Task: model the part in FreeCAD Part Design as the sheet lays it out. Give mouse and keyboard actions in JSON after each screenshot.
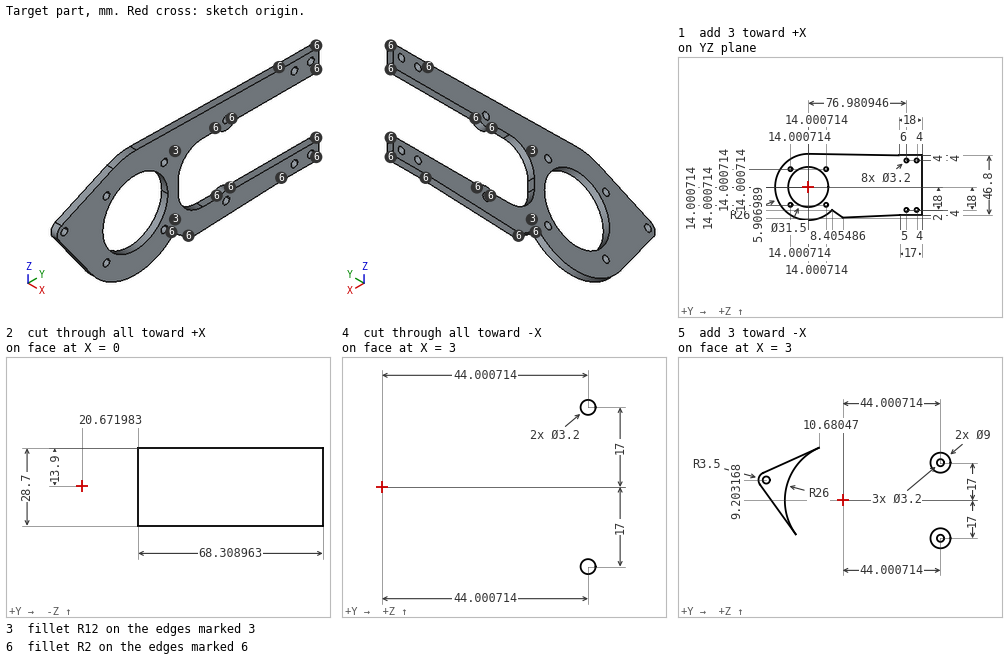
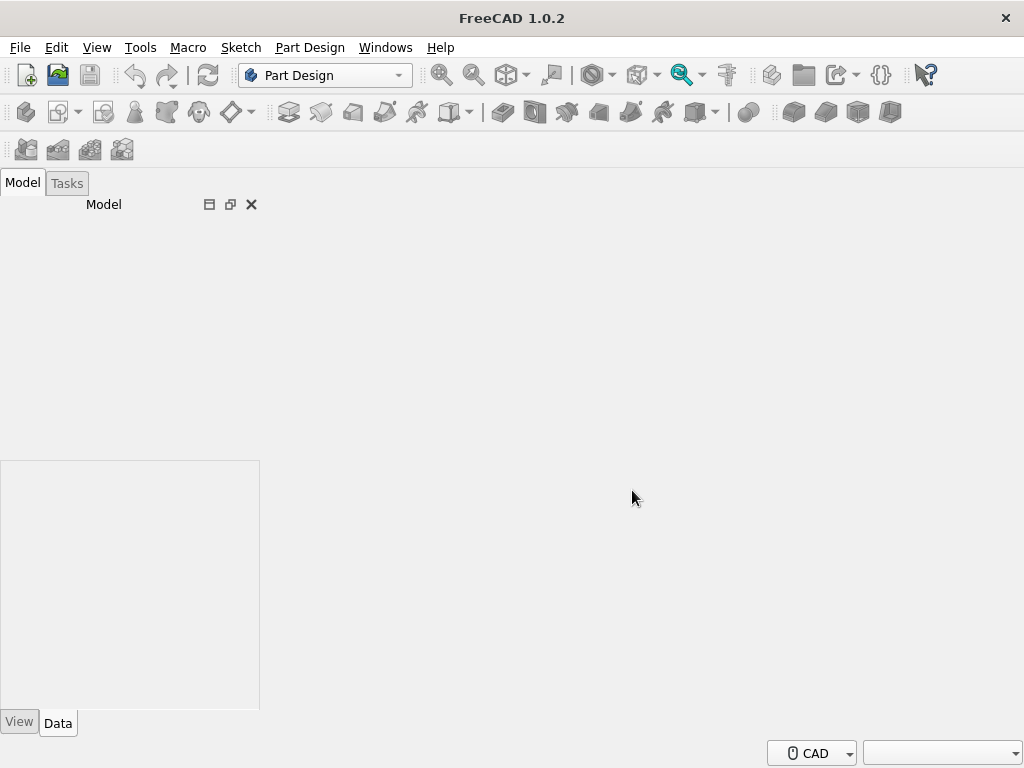
{"action": "left_click", "coordinate": [26, 76]}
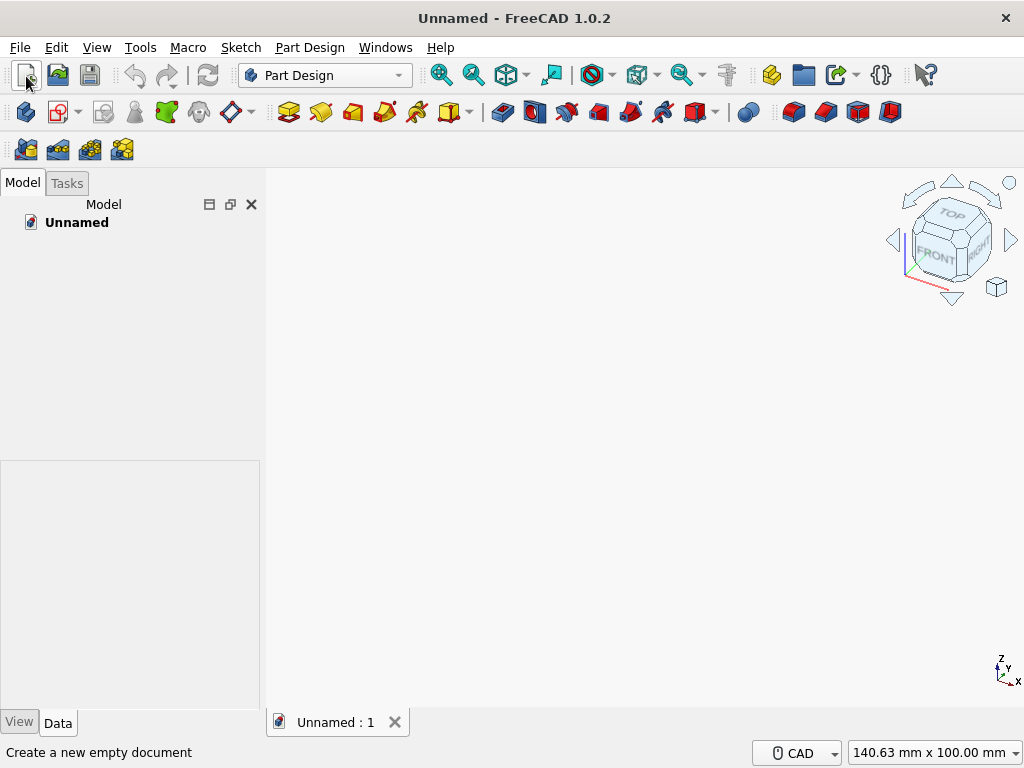
{"action": "left_click", "coordinate": [58, 112]}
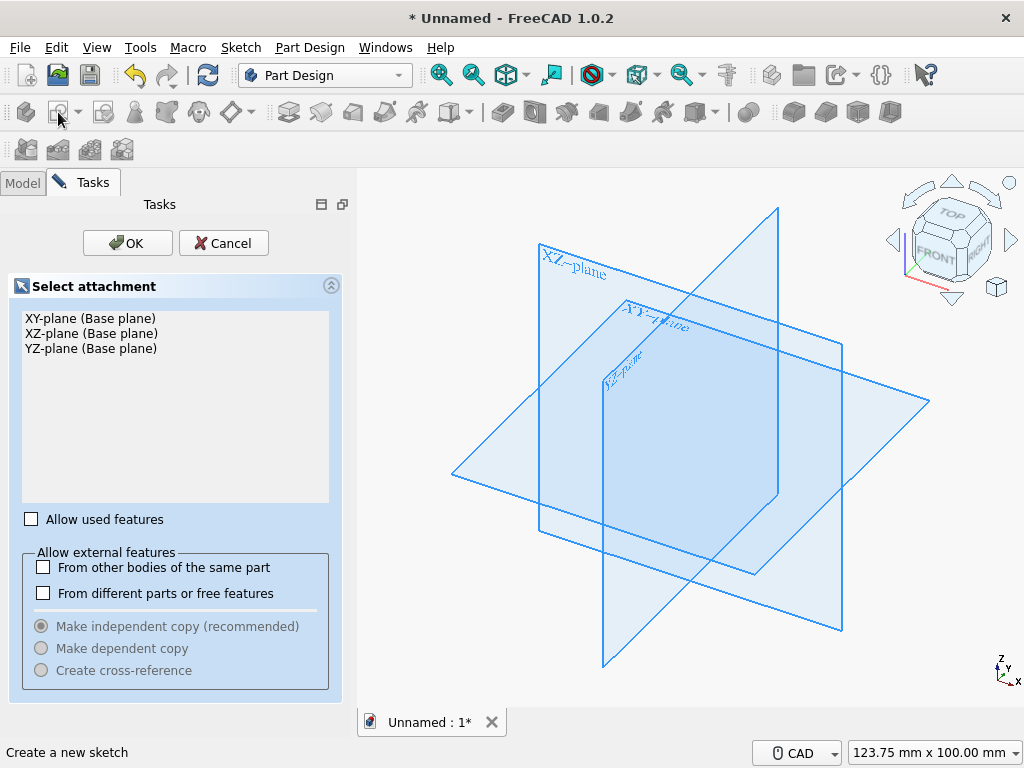
{"action": "left_click", "coordinate": [82, 348]}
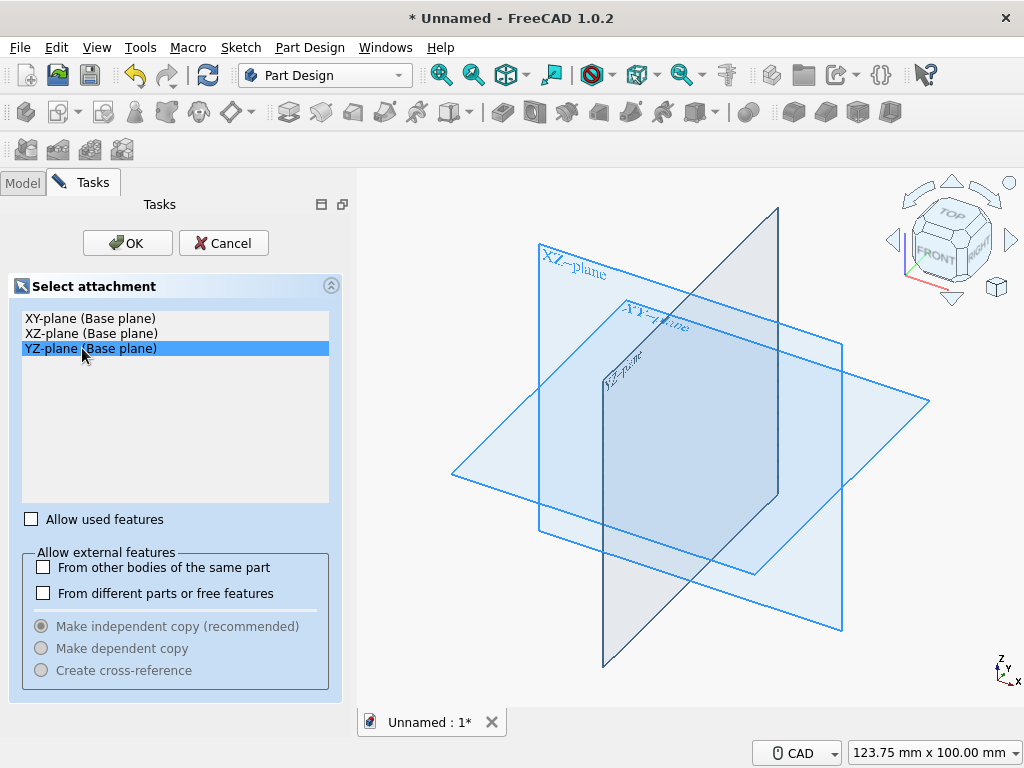
{"action": "left_click", "coordinate": [128, 243]}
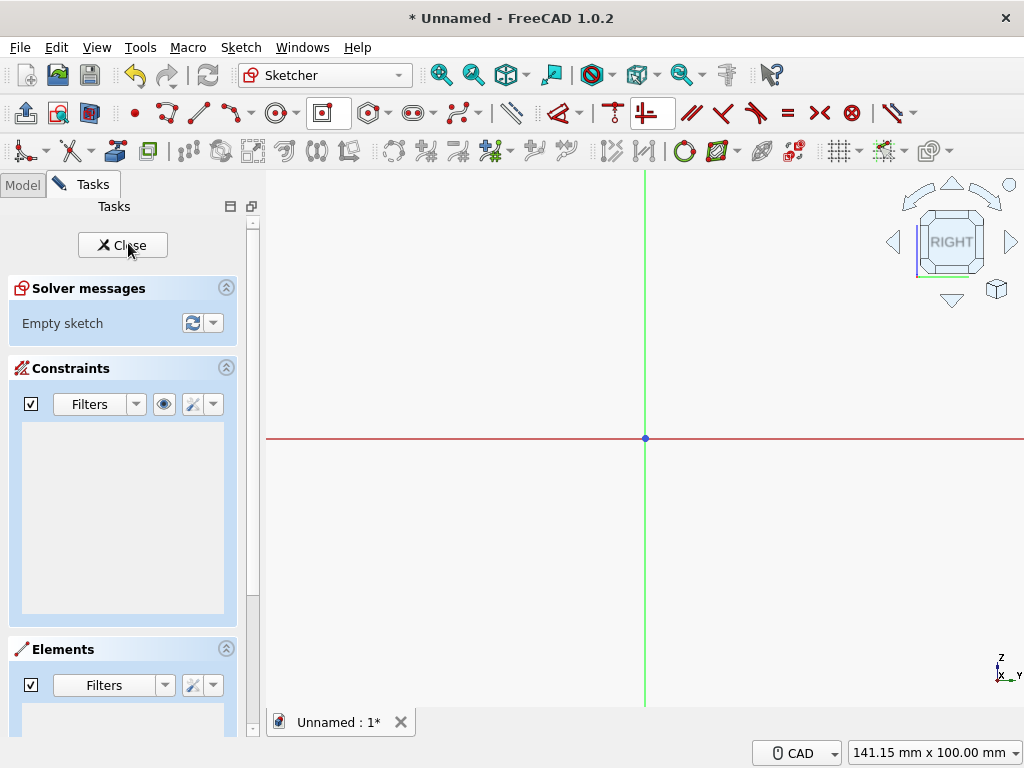
{"action": "scroll", "coordinate": [294, 445], "scroll_direction": "down", "scroll_amount": 3}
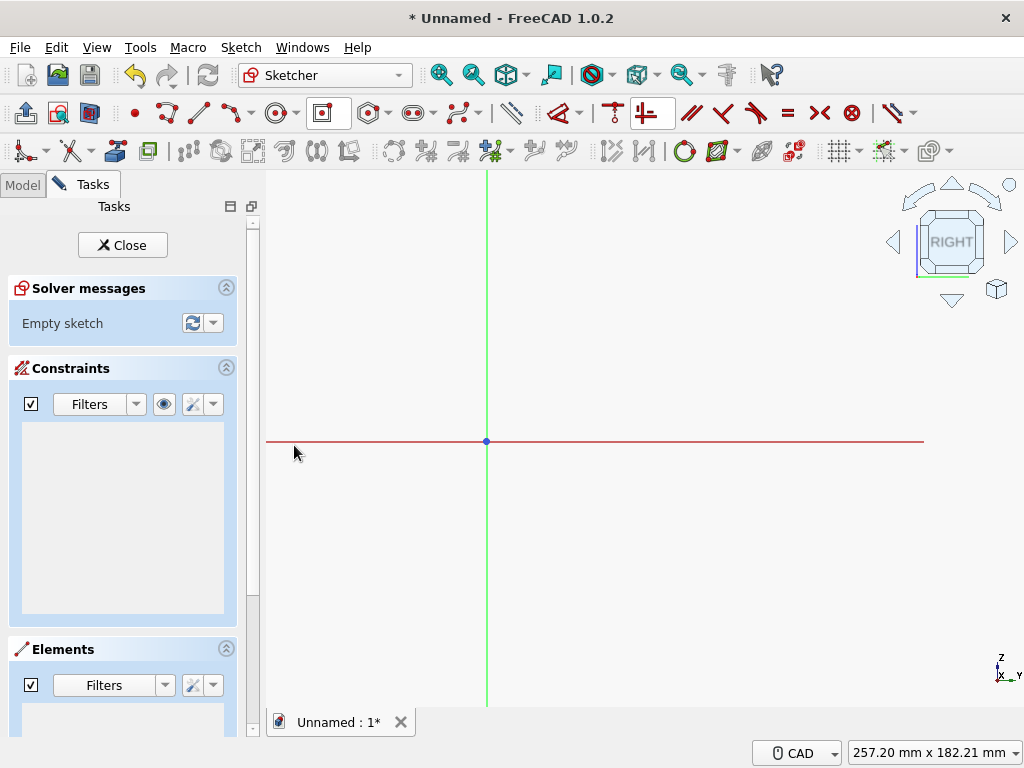
{"action": "left_click", "coordinate": [168, 114]}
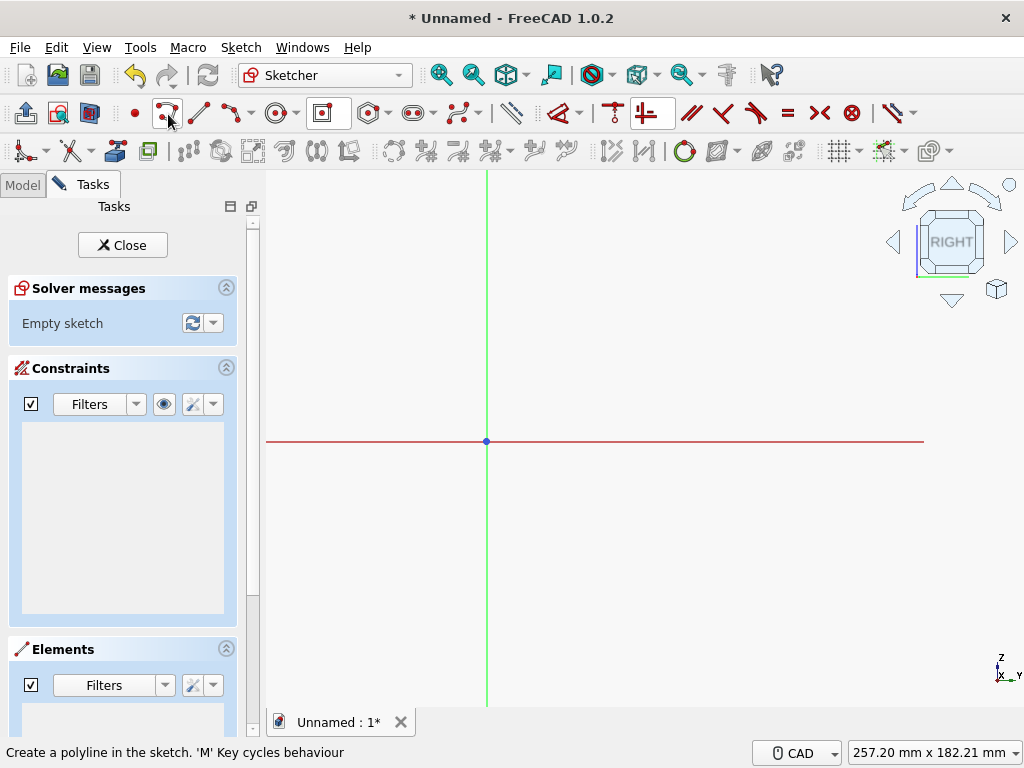
{"action": "left_click", "coordinate": [542, 495]}
{"action": "left_click", "coordinate": [566, 512]}
{"action": "left_click", "coordinate": [699, 505]}
{"action": "left_click", "coordinate": [749, 505]}
{"action": "left_click", "coordinate": [749, 369]}
{"action": "left_click", "coordinate": [696, 369]}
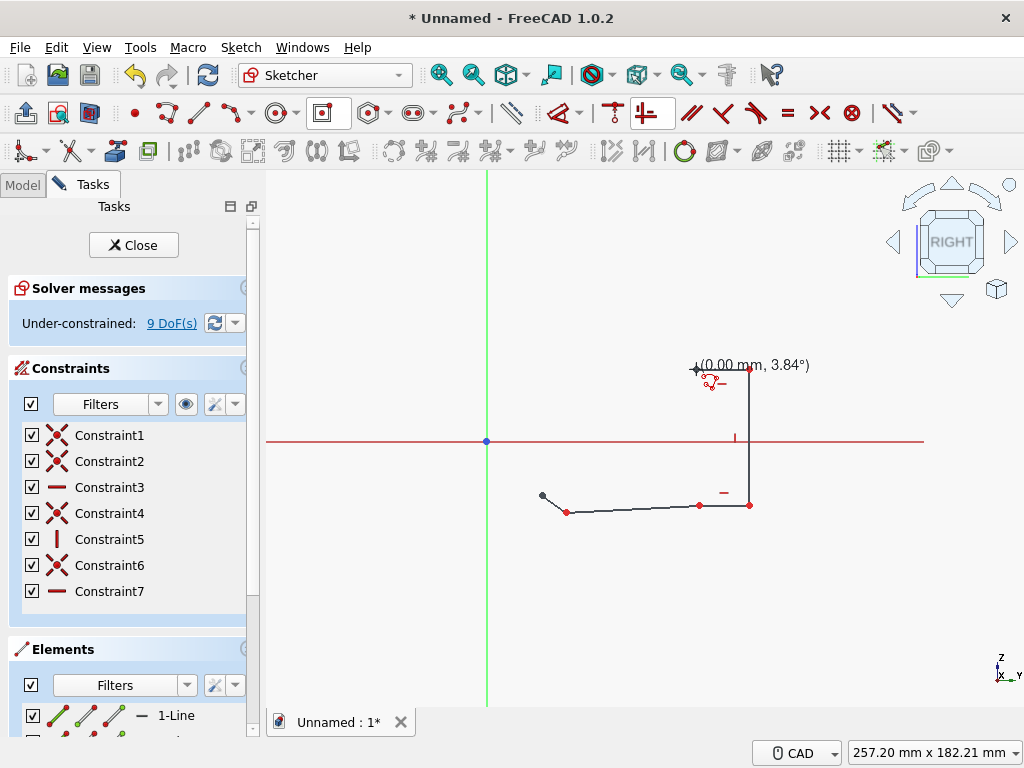
{"action": "scroll", "coordinate": [488, 365], "scroll_direction": "up", "scroll_amount": 13}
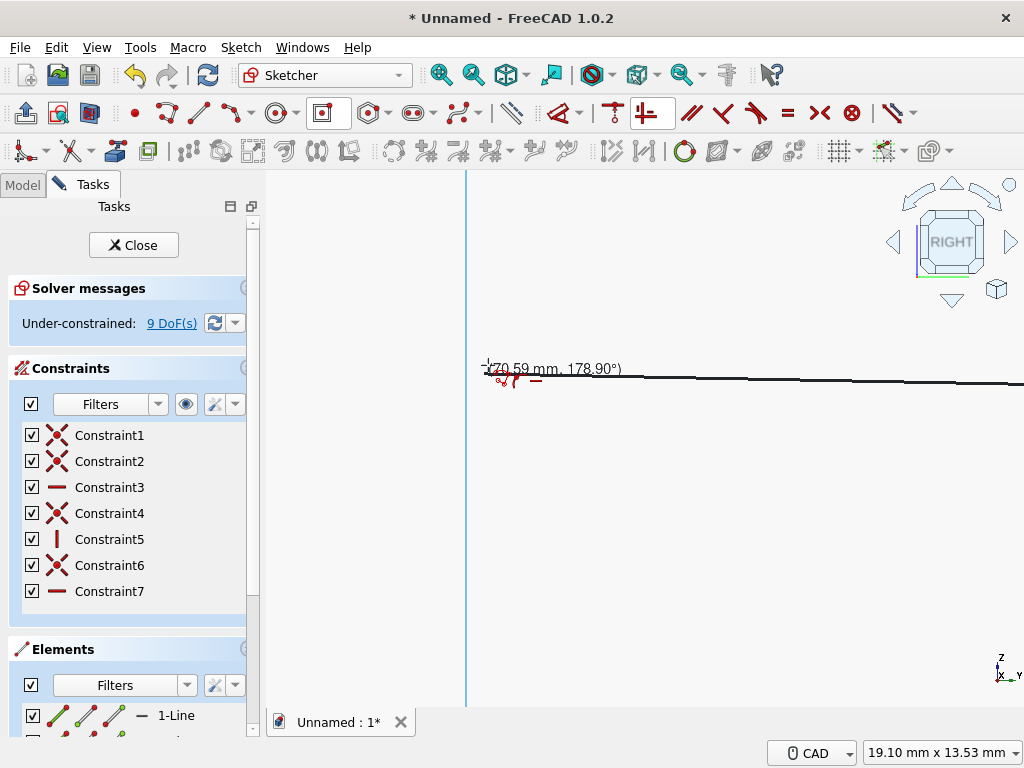
{"action": "left_click", "coordinate": [484, 287]}
{"action": "right_click", "coordinate": [484, 287]}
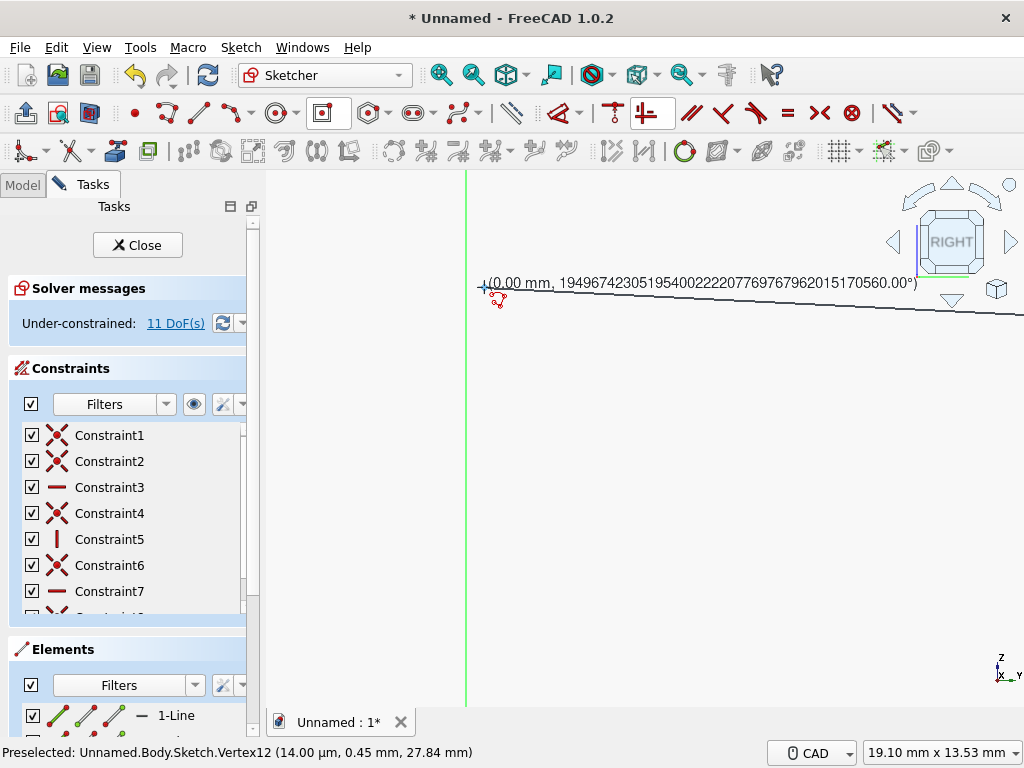
{"action": "left_click", "coordinate": [232, 114]}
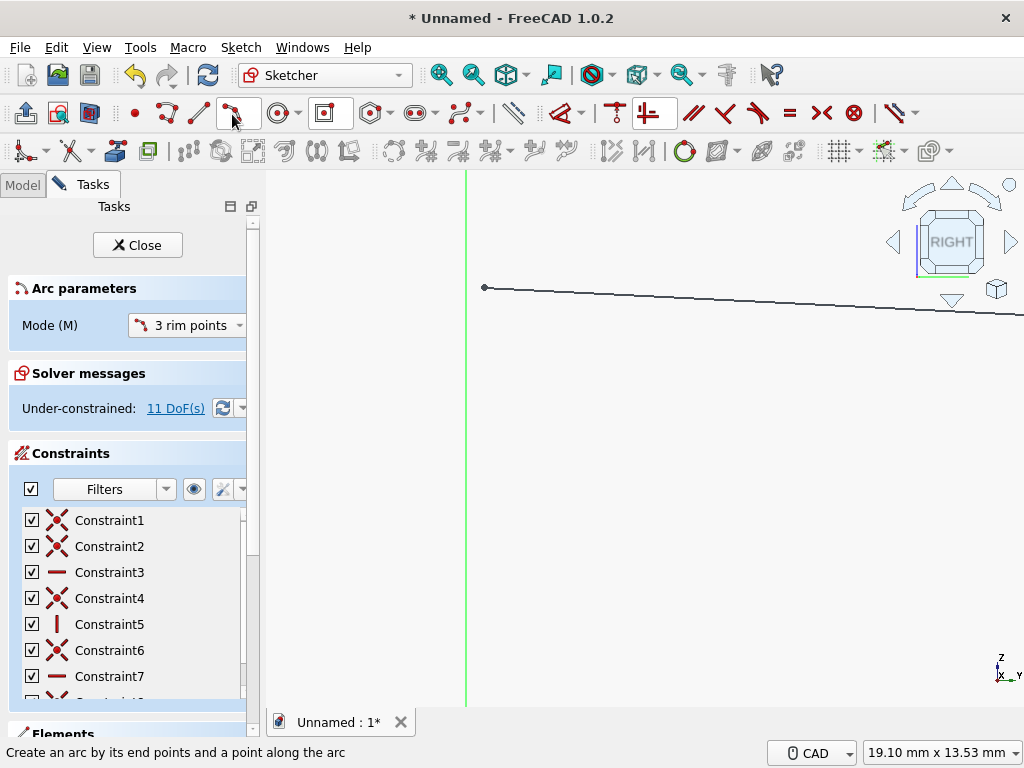
{"action": "left_click", "coordinate": [484, 288]}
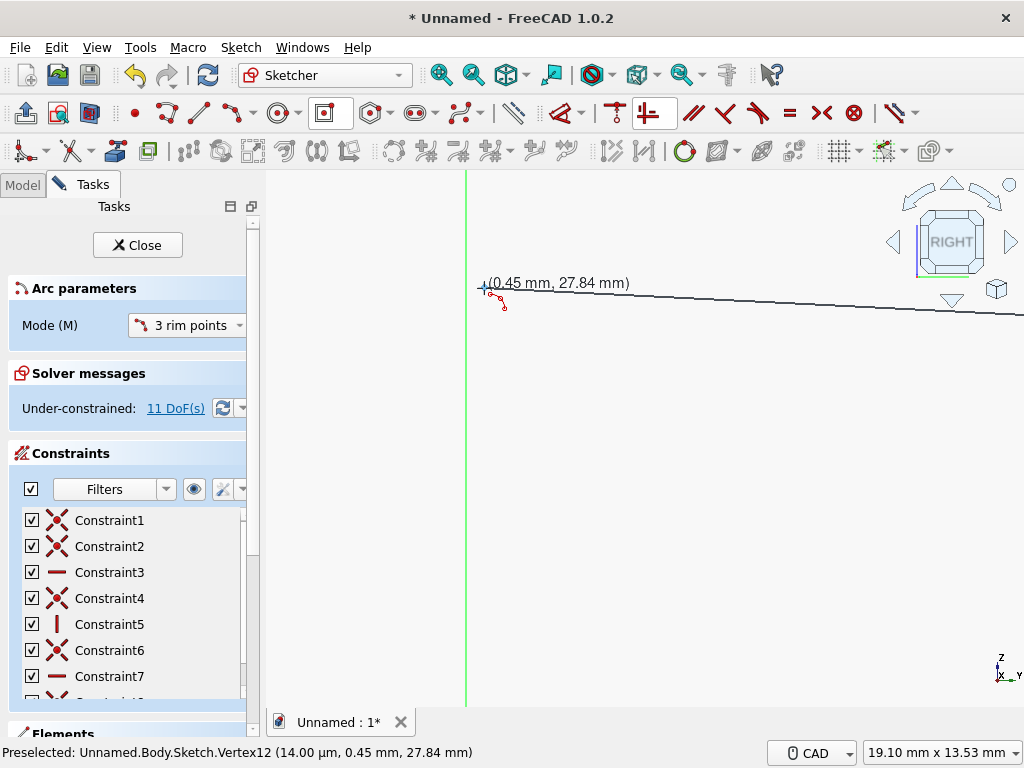
{"action": "scroll", "coordinate": [459, 347], "scroll_direction": "down", "scroll_amount": 12}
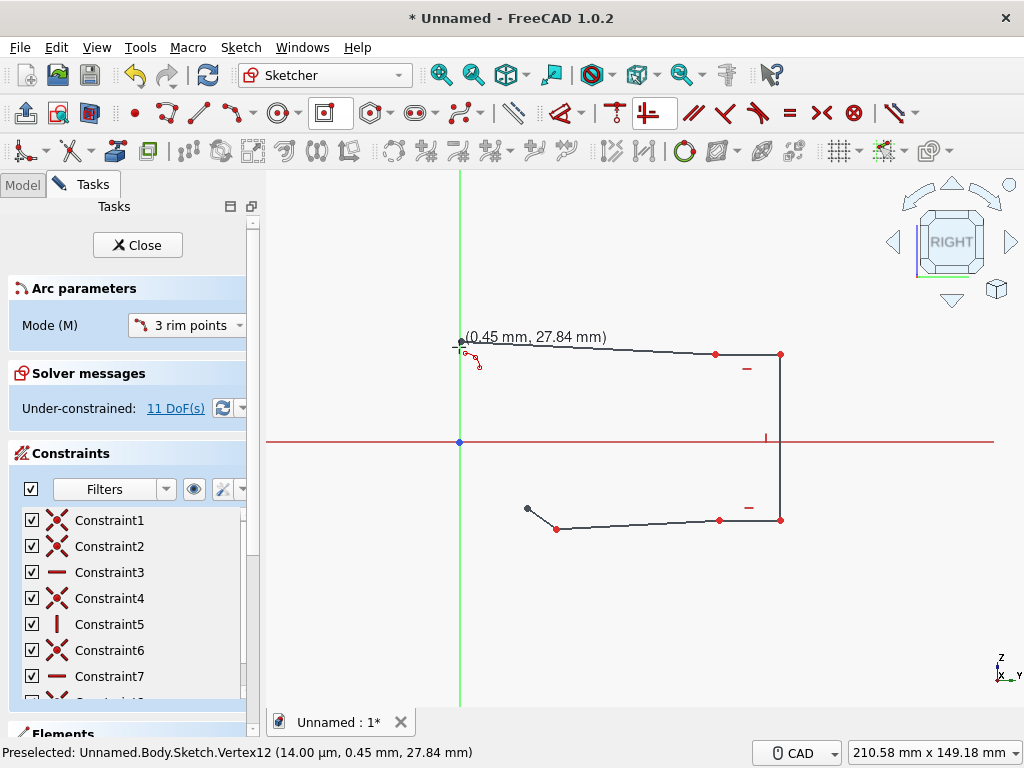
{"action": "left_click", "coordinate": [527, 509]}
{"action": "left_click", "coordinate": [373, 478]}